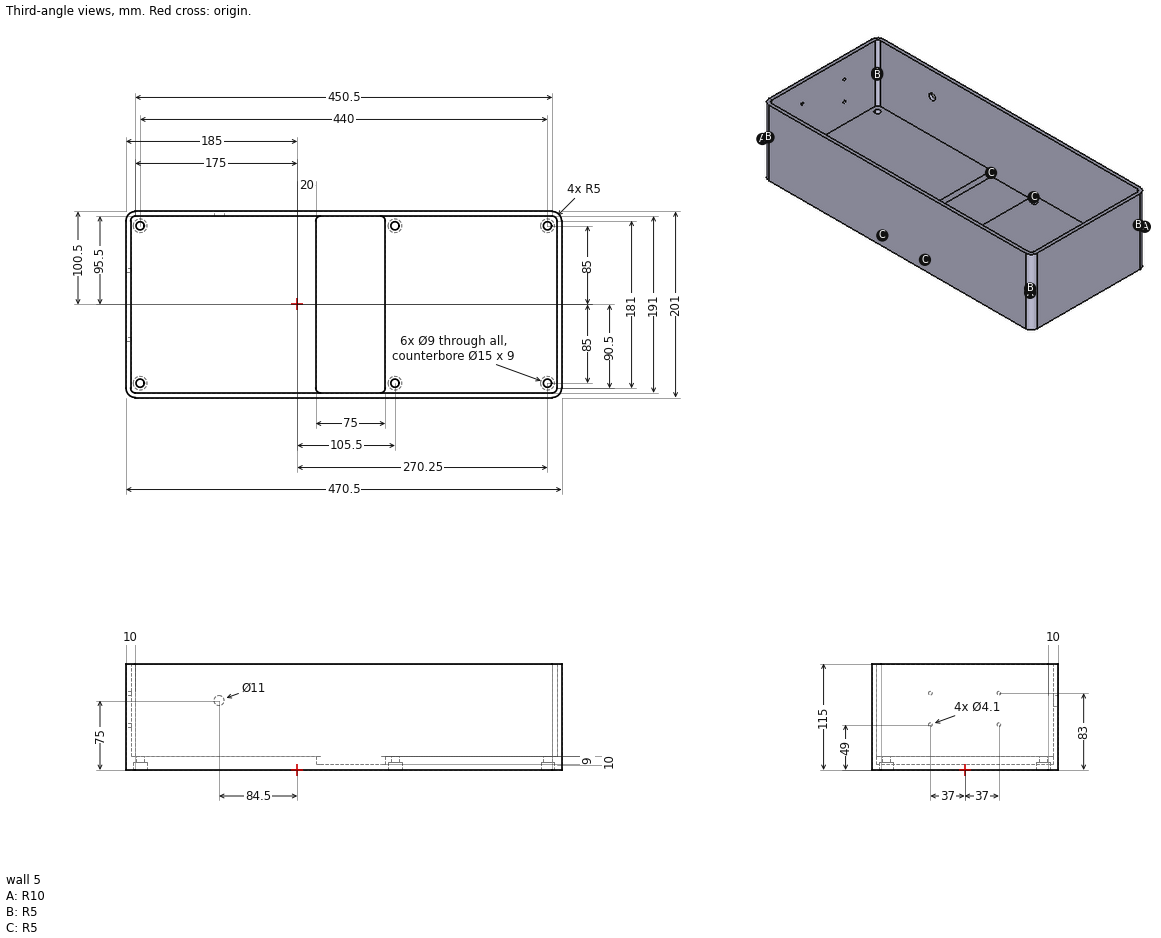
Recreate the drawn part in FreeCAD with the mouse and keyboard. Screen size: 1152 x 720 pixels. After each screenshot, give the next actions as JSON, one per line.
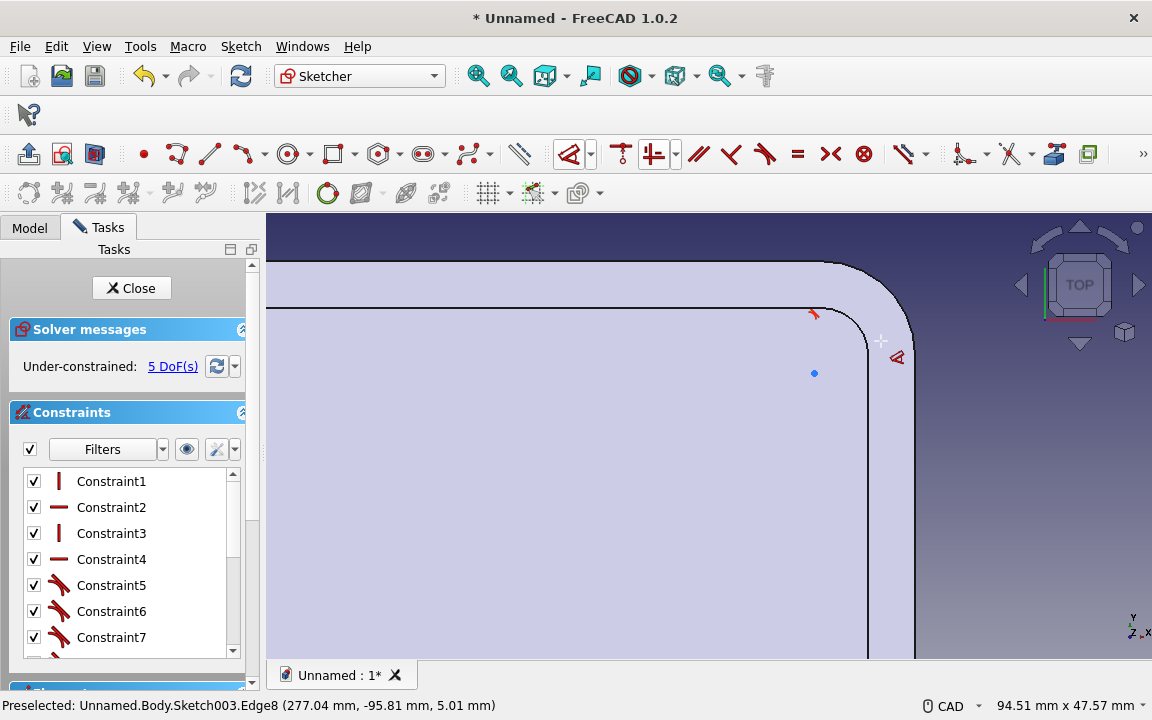
{"action": "left_click", "coordinate": [879, 341]}
{"action": "left_click", "coordinate": [907, 326]}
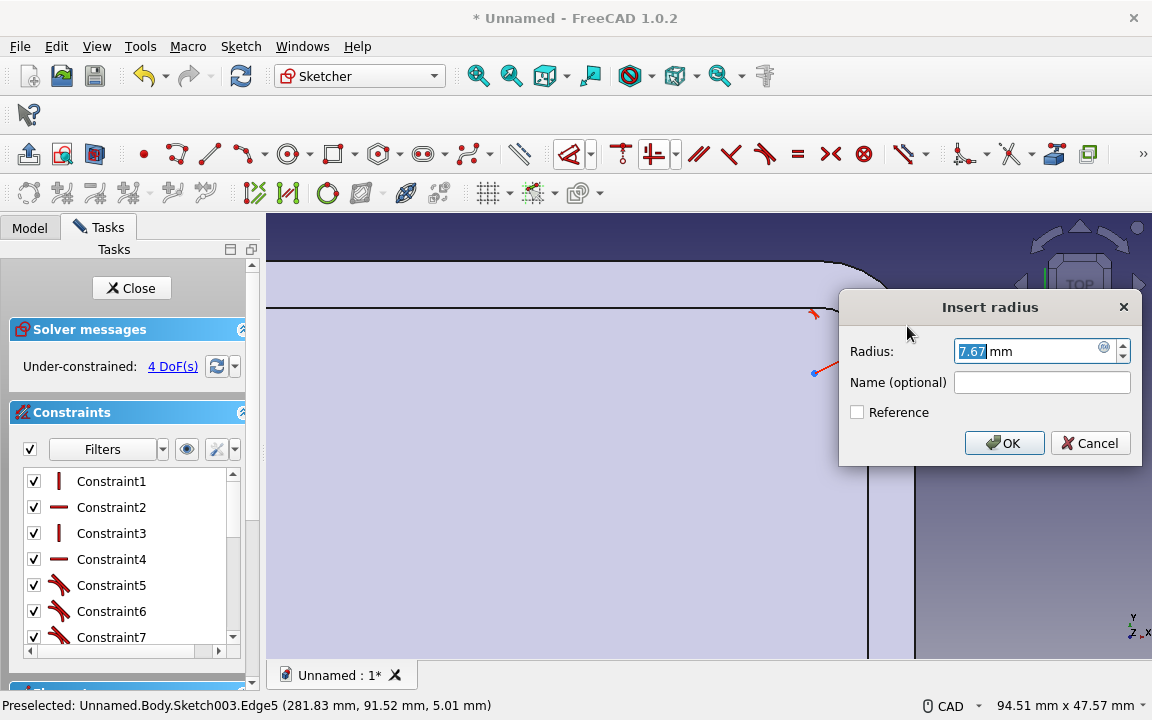
{"action": "type", "text": "5"}
{"action": "key", "text": "Return"}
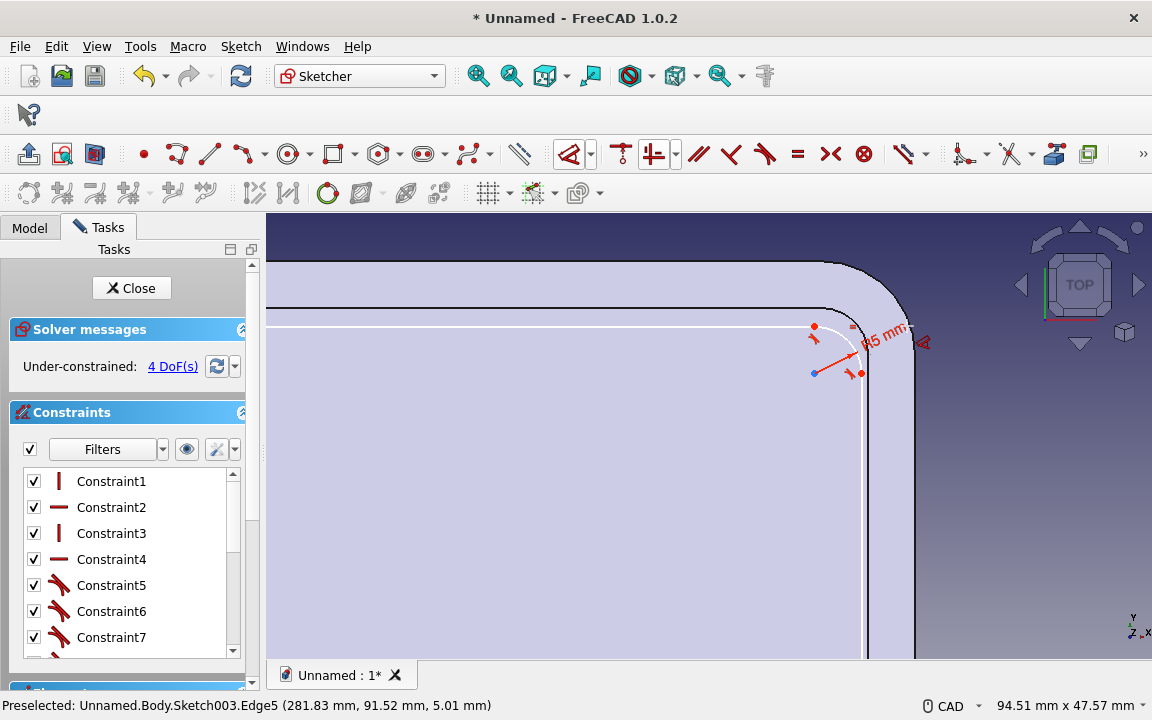
{"action": "scroll", "coordinate": [881, 340], "scroll_direction": "down", "scroll_amount": 11}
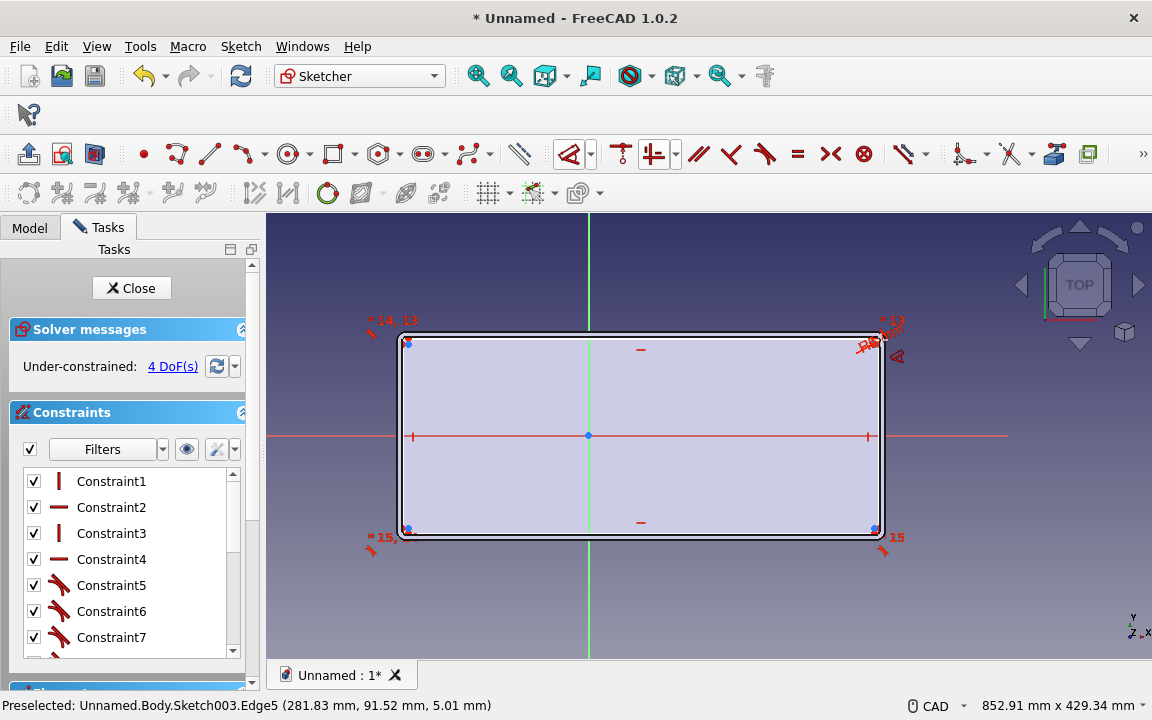
{"action": "left_click", "coordinate": [879, 473]}
{"action": "left_click", "coordinate": [913, 394]}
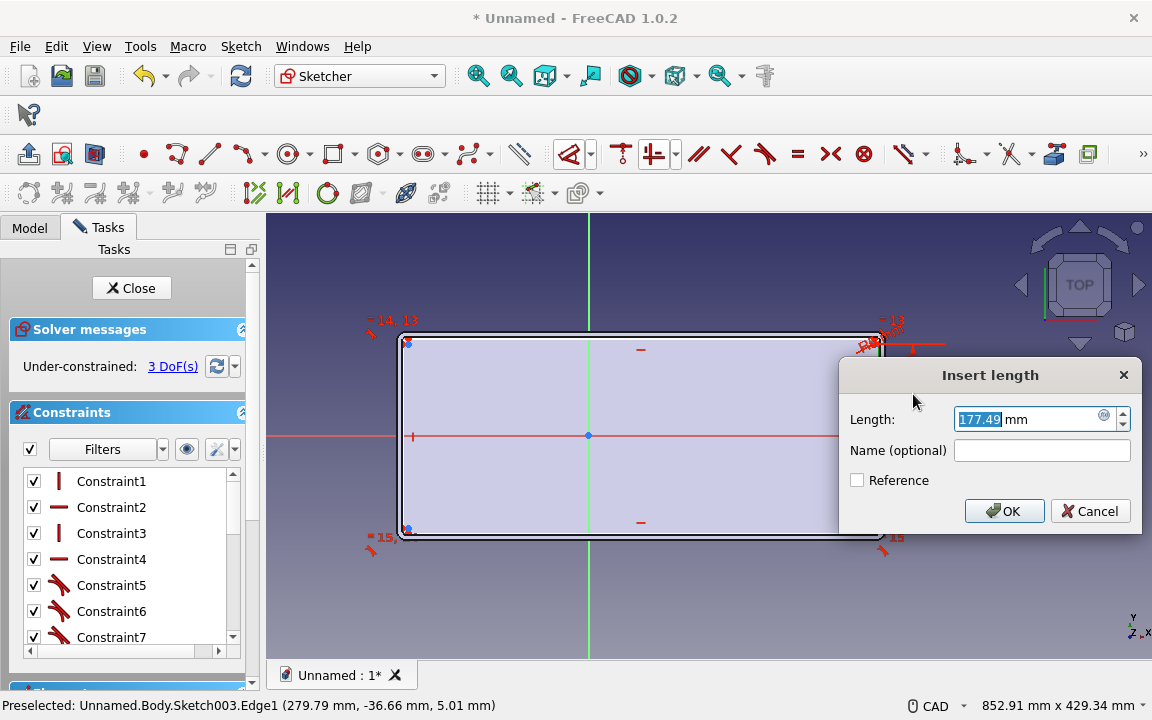
{"action": "type", "text": "181"}
{"action": "key", "text": "Return"}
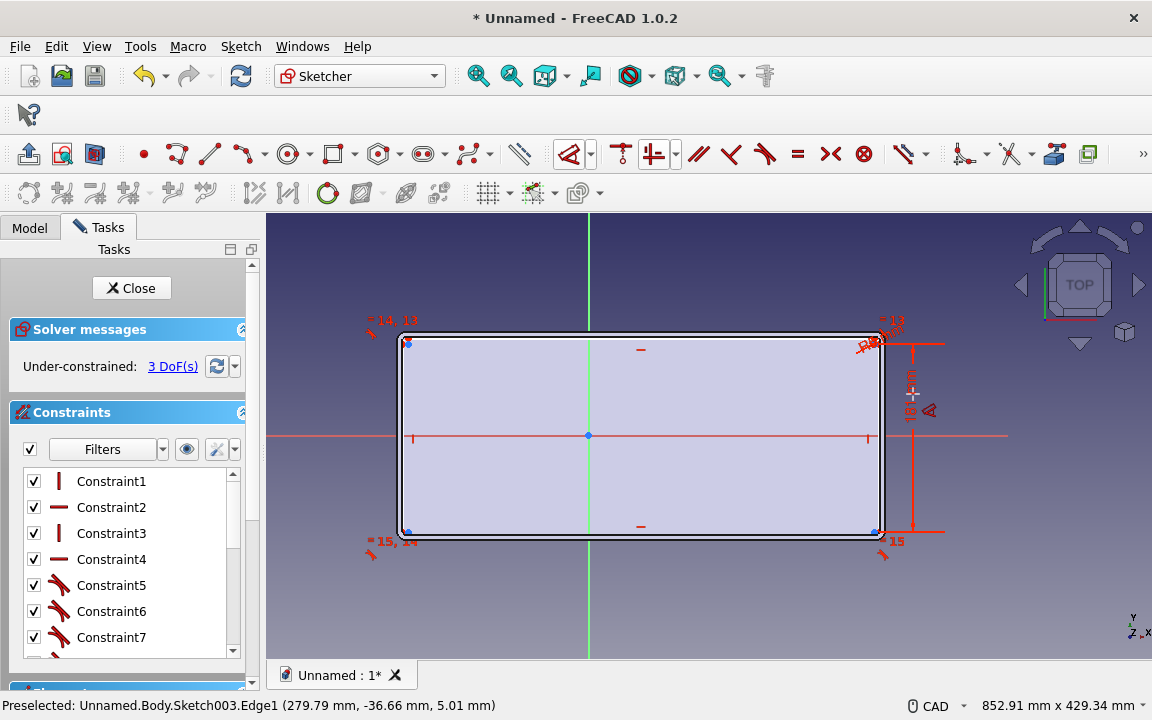
{"action": "scroll", "coordinate": [408, 339], "scroll_direction": "up", "scroll_amount": 5}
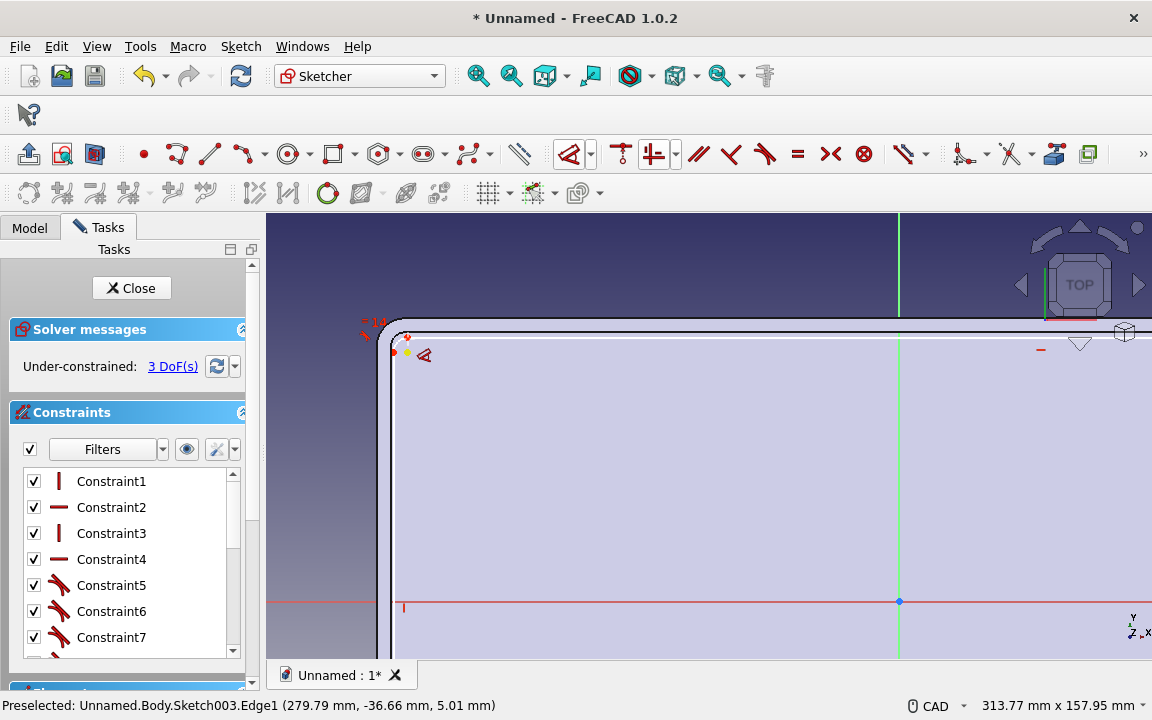
{"action": "left_click", "coordinate": [408, 338]}
{"action": "left_click", "coordinate": [654, 304]}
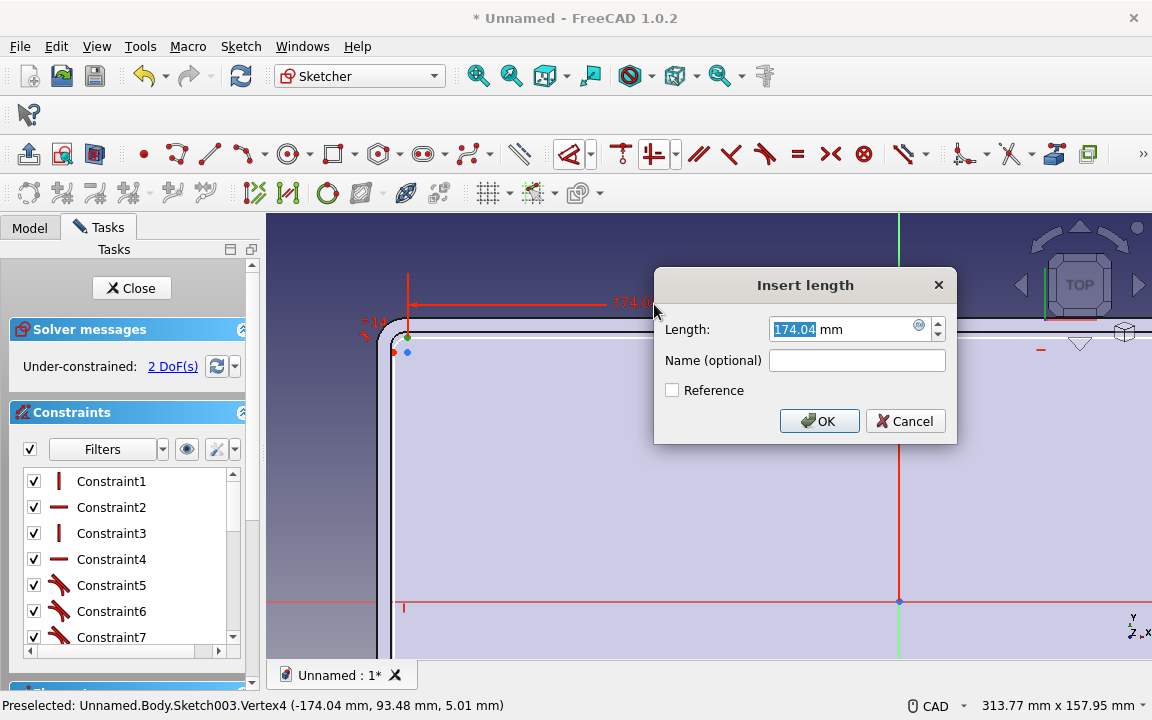
{"action": "type", "text": "175"}
{"action": "key", "text": "Return"}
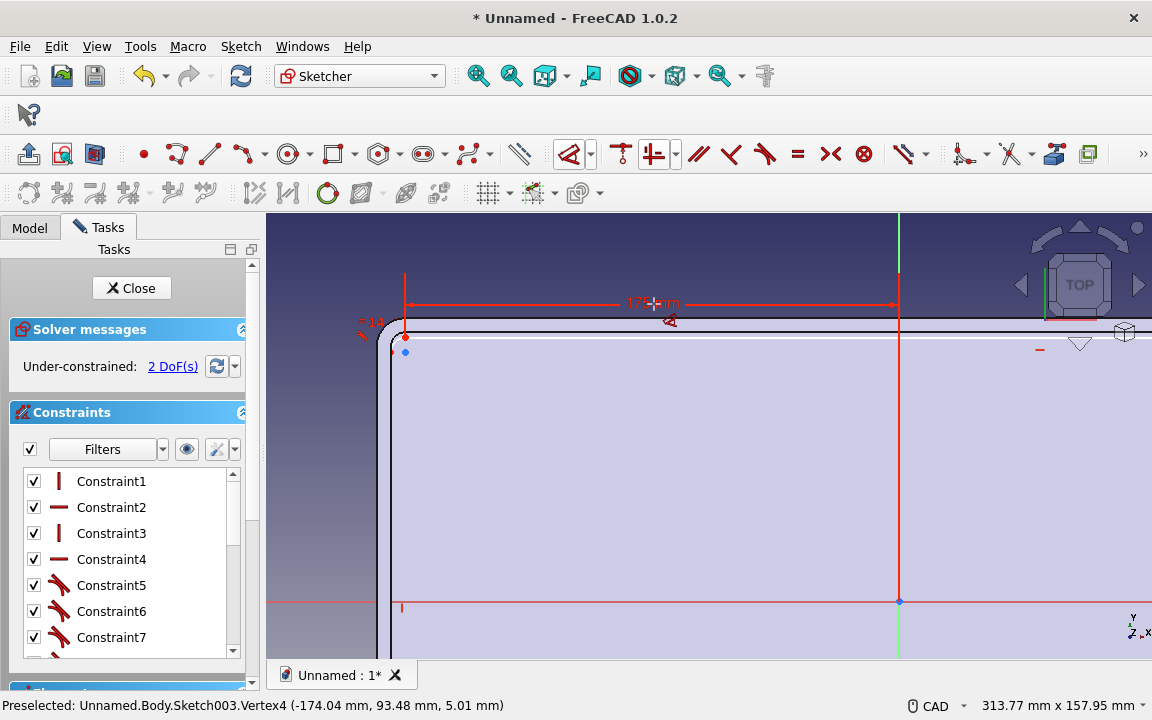
{"action": "left_click", "coordinate": [786, 338]}
{"action": "left_click", "coordinate": [562, 304]}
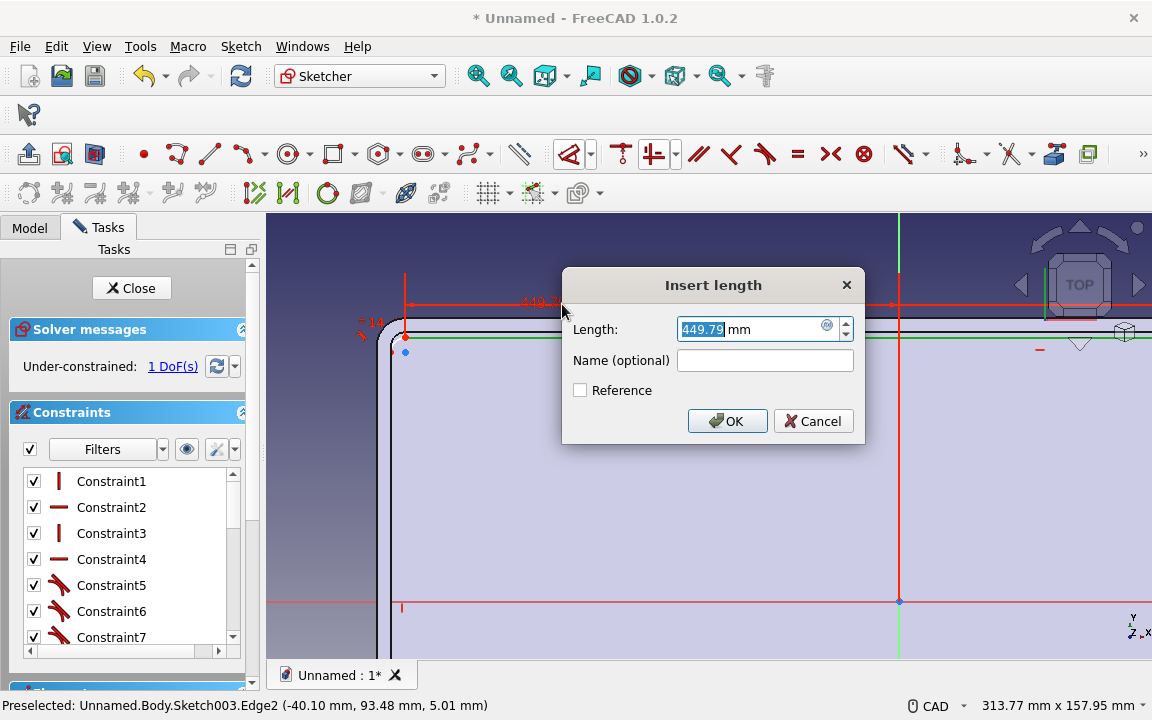
{"action": "type", "text": "450.5"}
{"action": "key", "text": "Return"}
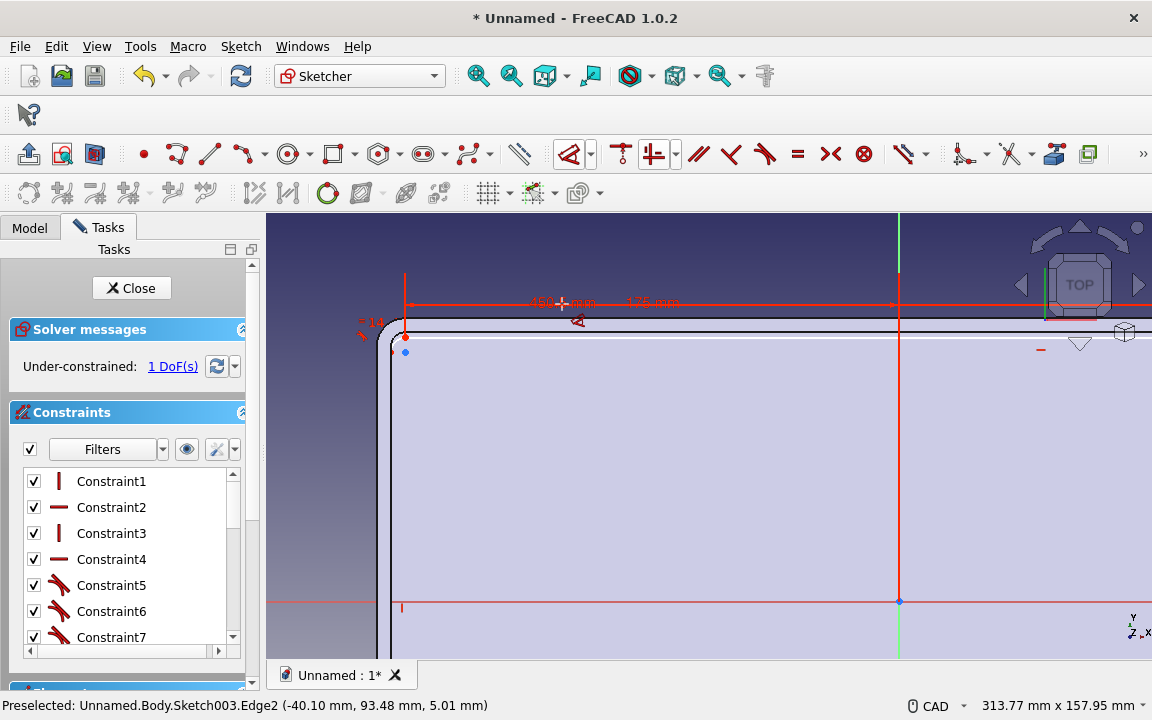
{"action": "scroll", "coordinate": [407, 339], "scroll_direction": "down", "scroll_amount": 5}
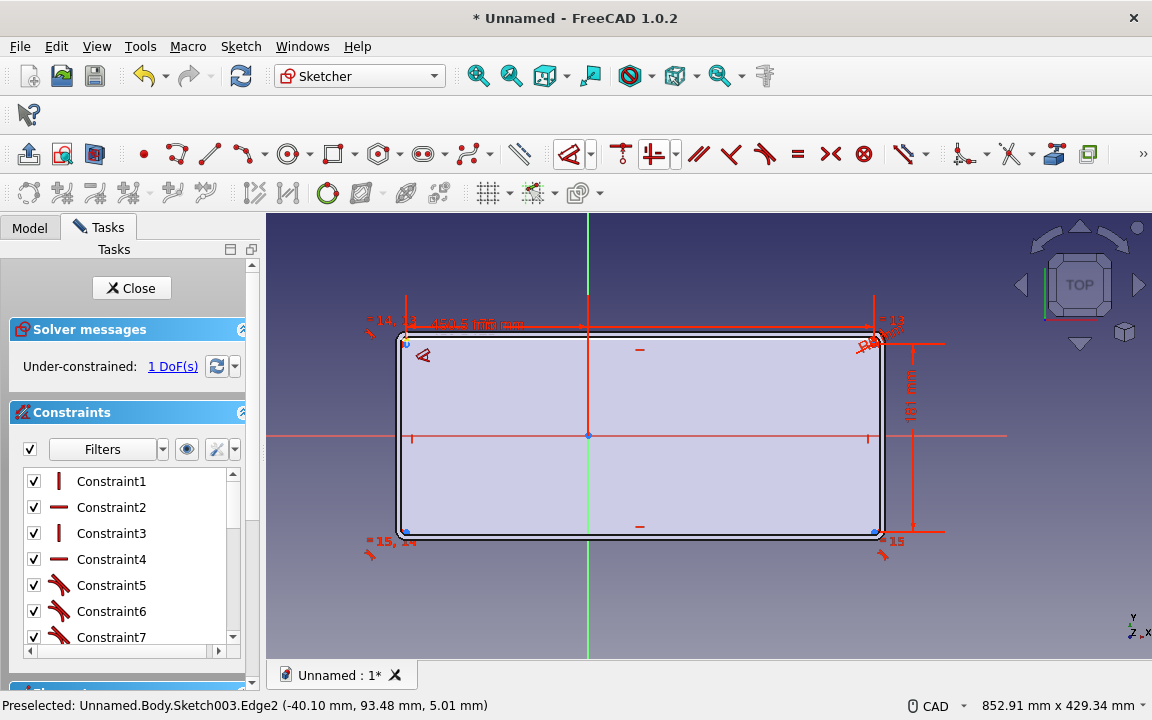
{"action": "scroll", "coordinate": [880, 532], "scroll_direction": "up", "scroll_amount": 5}